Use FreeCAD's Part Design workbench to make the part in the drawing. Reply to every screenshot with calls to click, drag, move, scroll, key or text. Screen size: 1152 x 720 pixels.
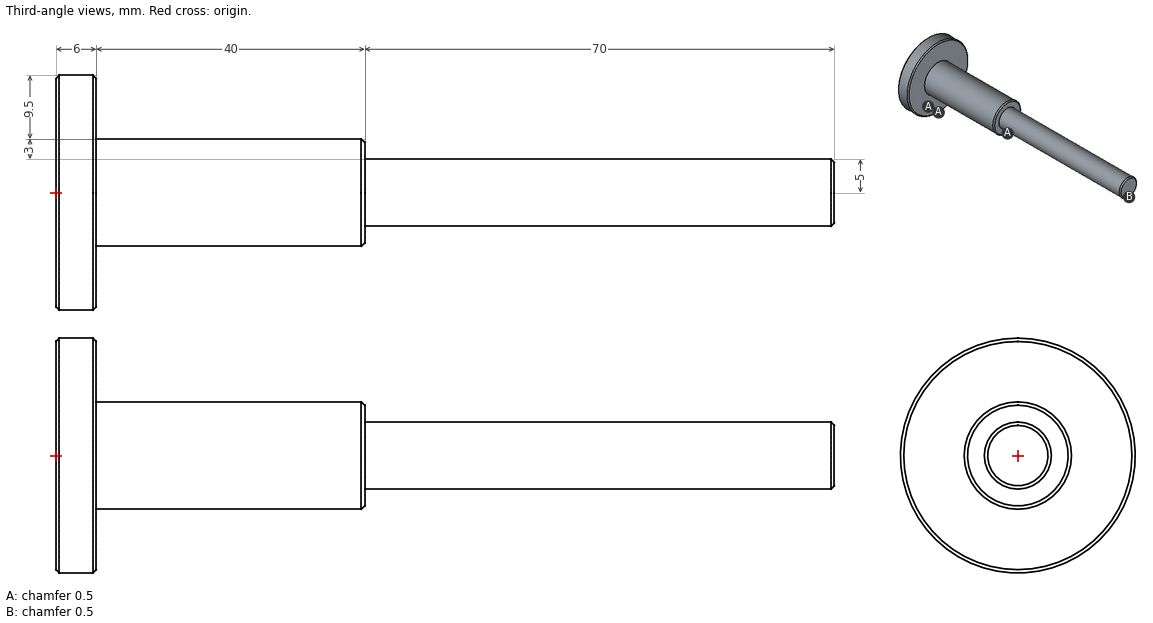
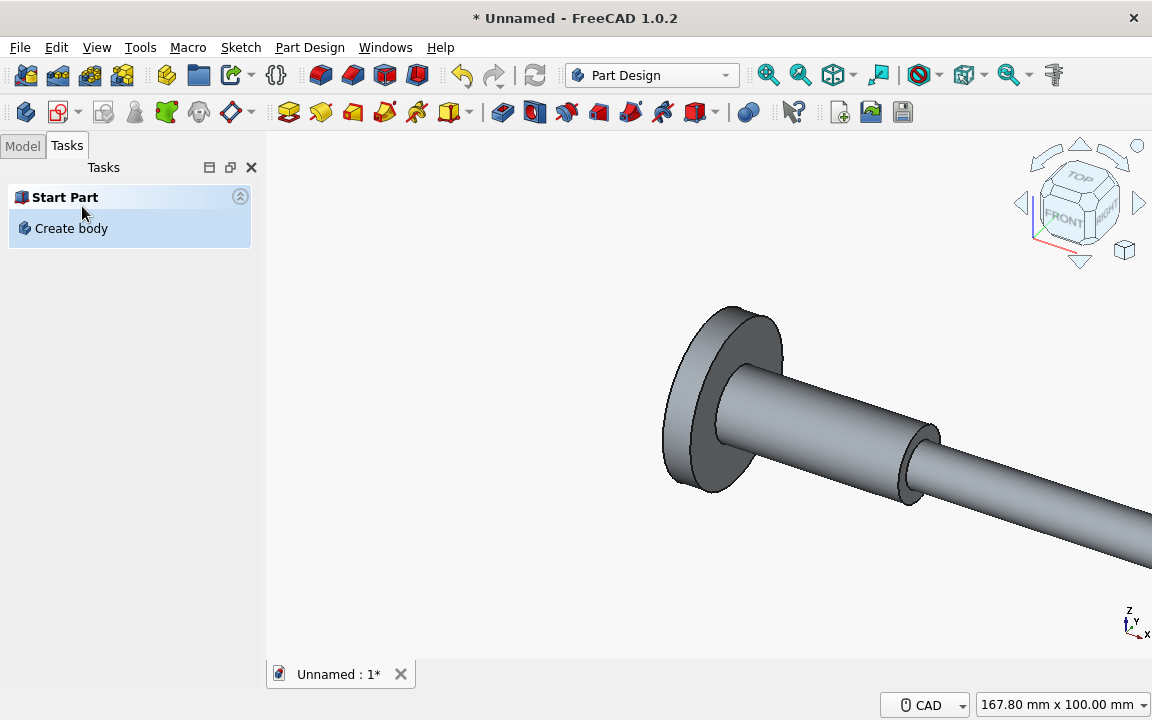
click(770, 76)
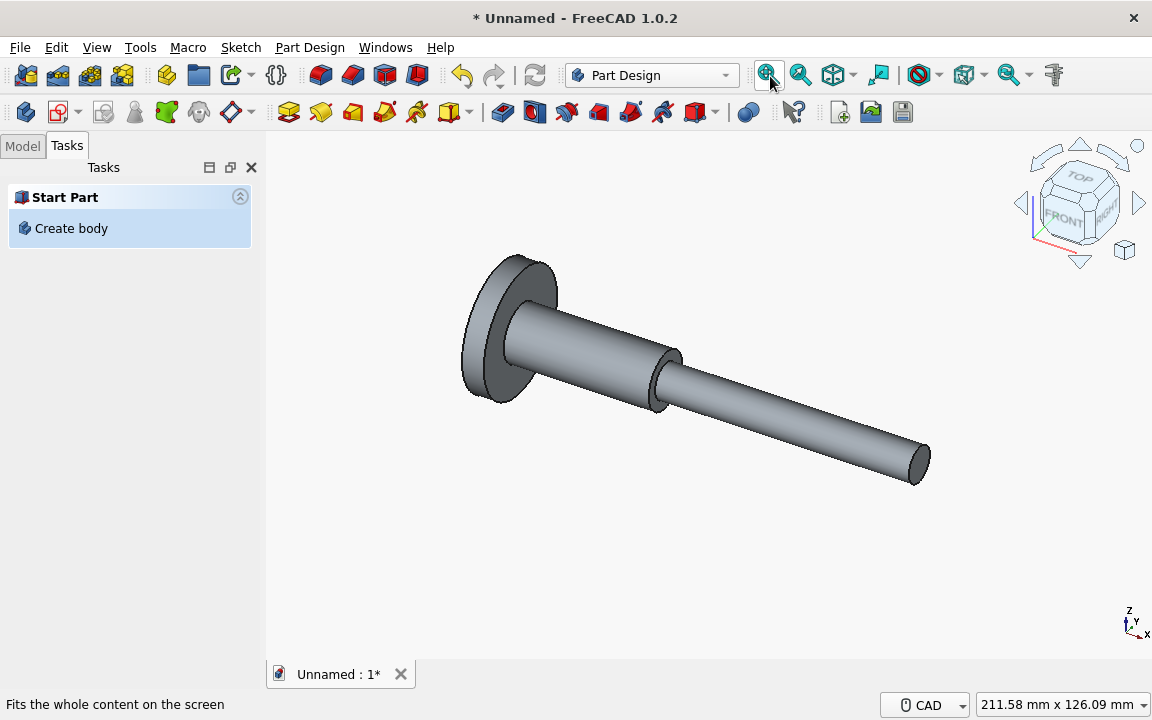
click(649, 396)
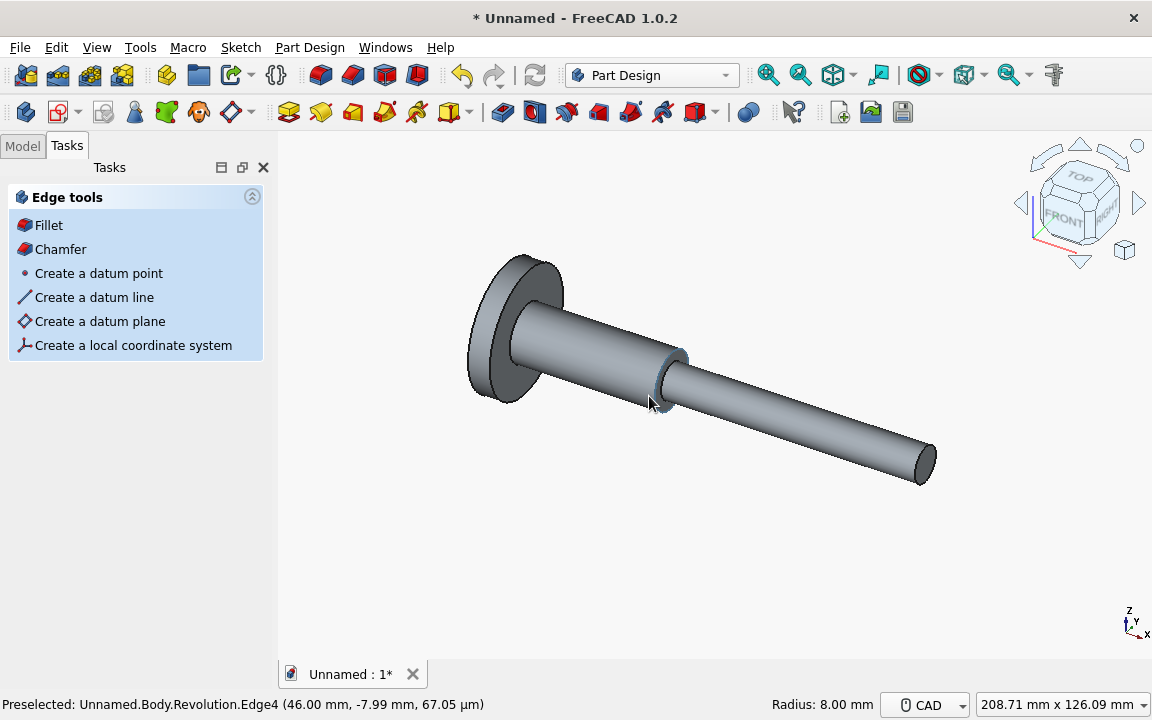
click(490, 368, ctrl)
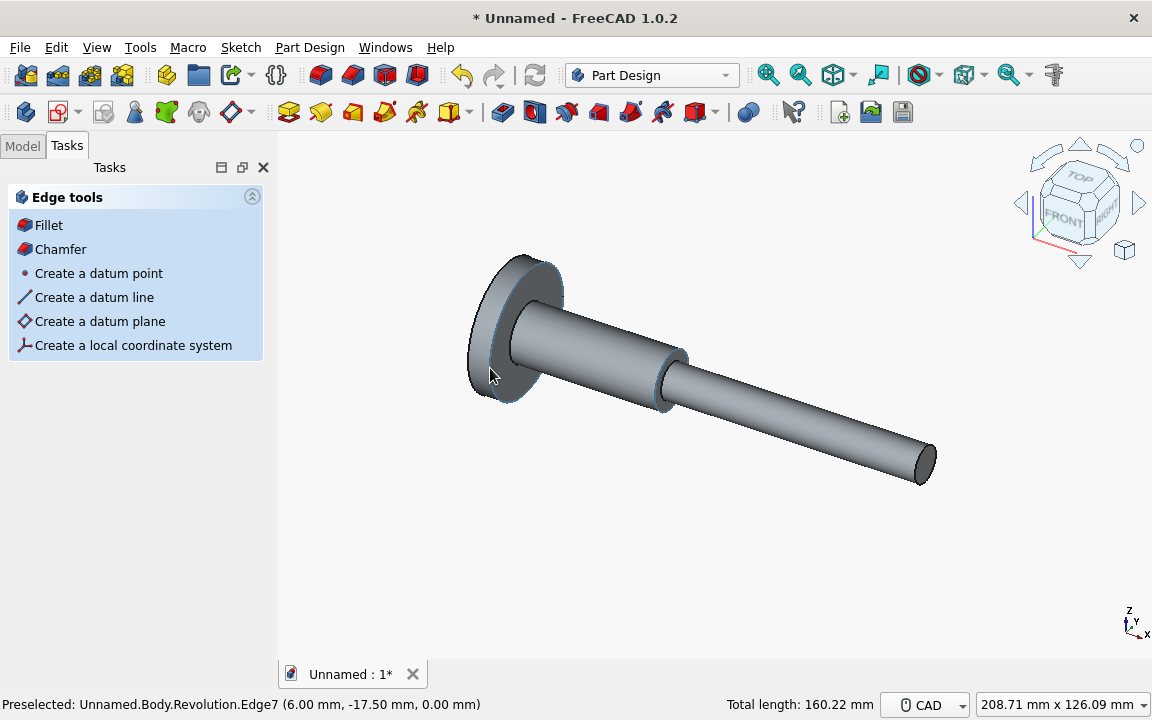
key(0)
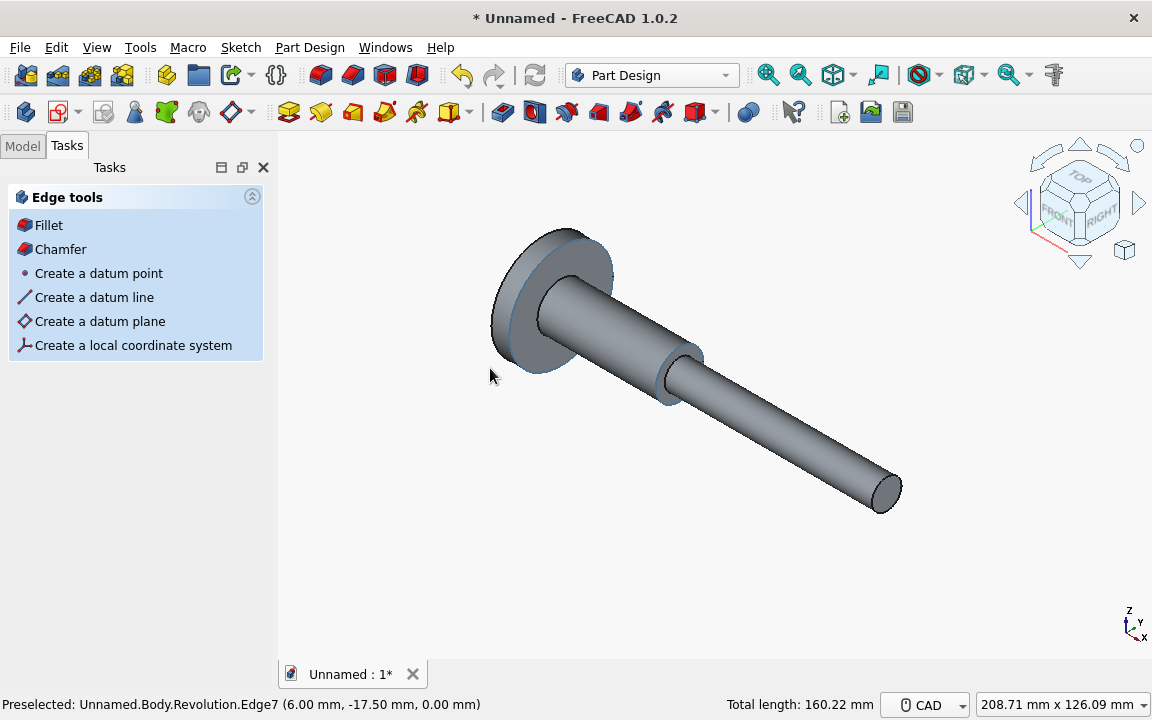
key(2)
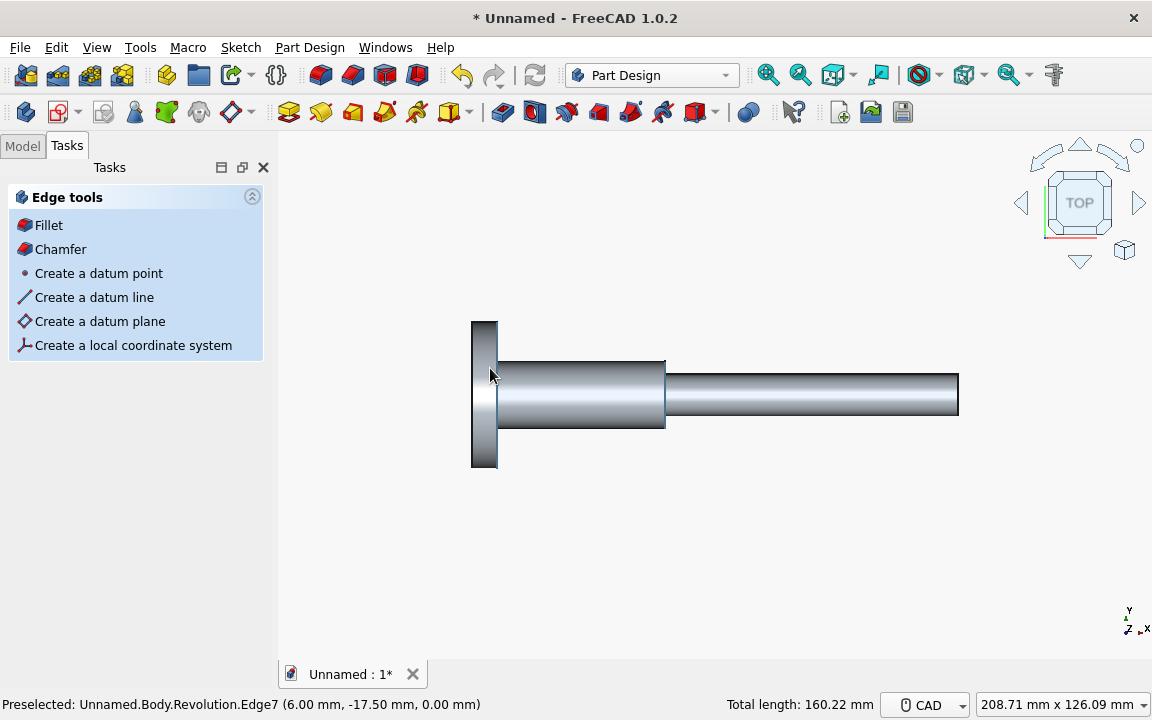
click(472, 453, ctrl)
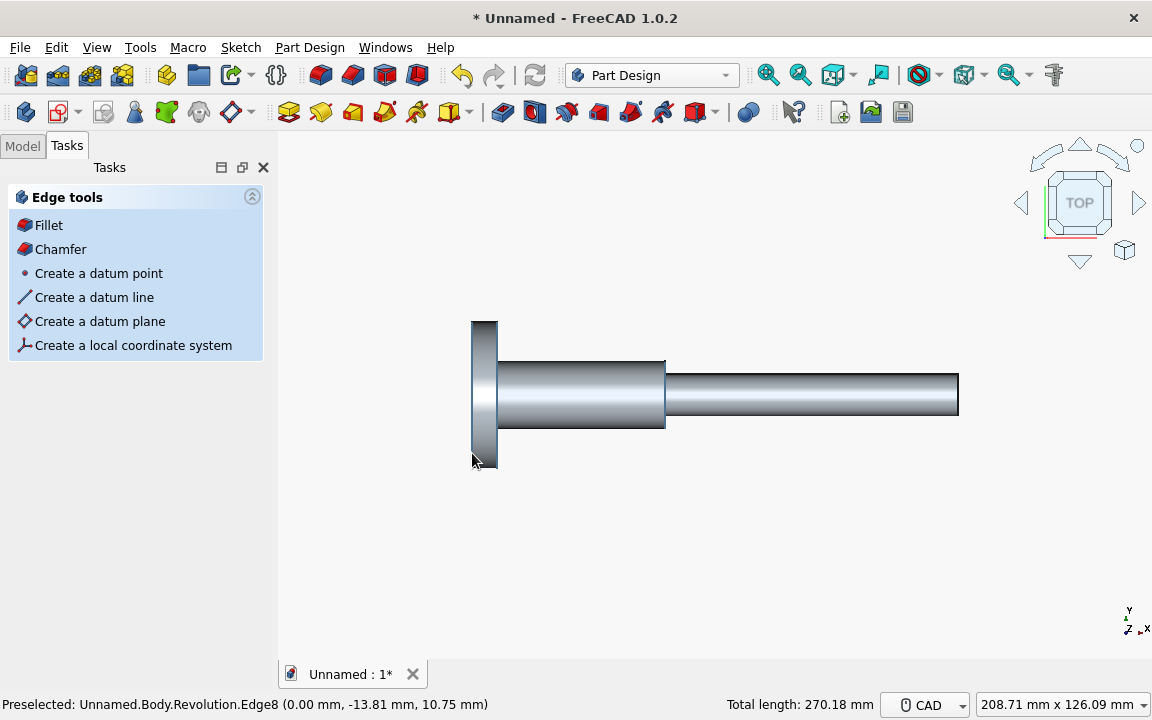
click(354, 76)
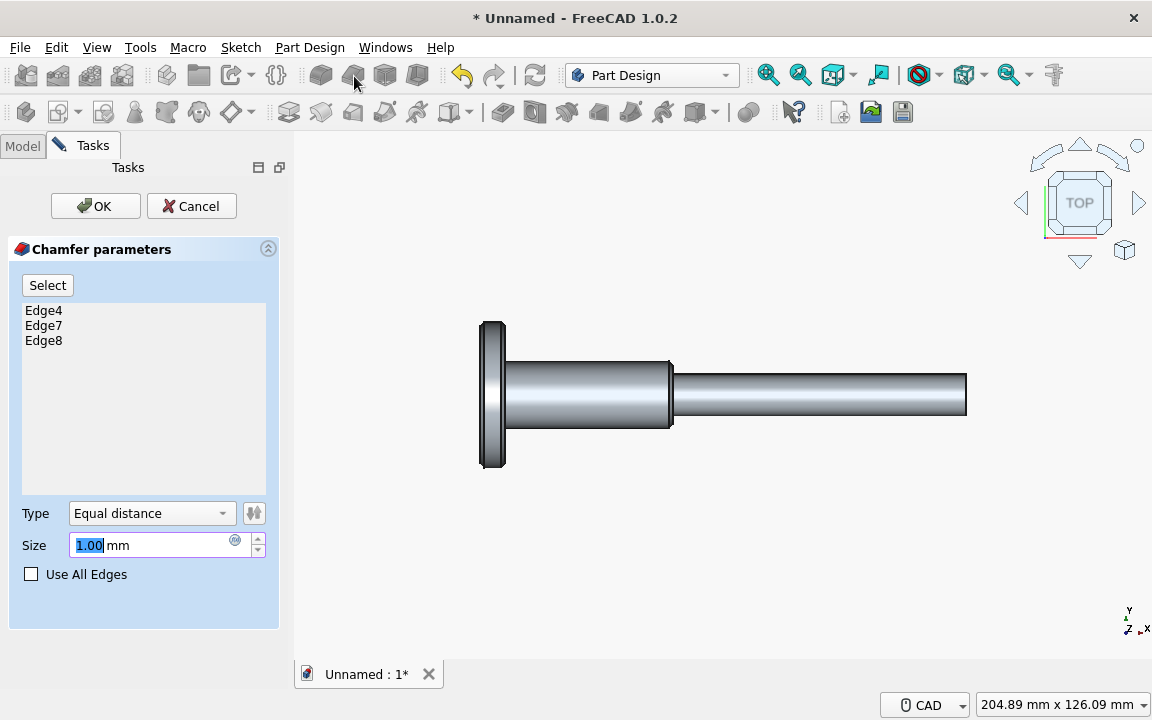
text(0.5)
key(Tab)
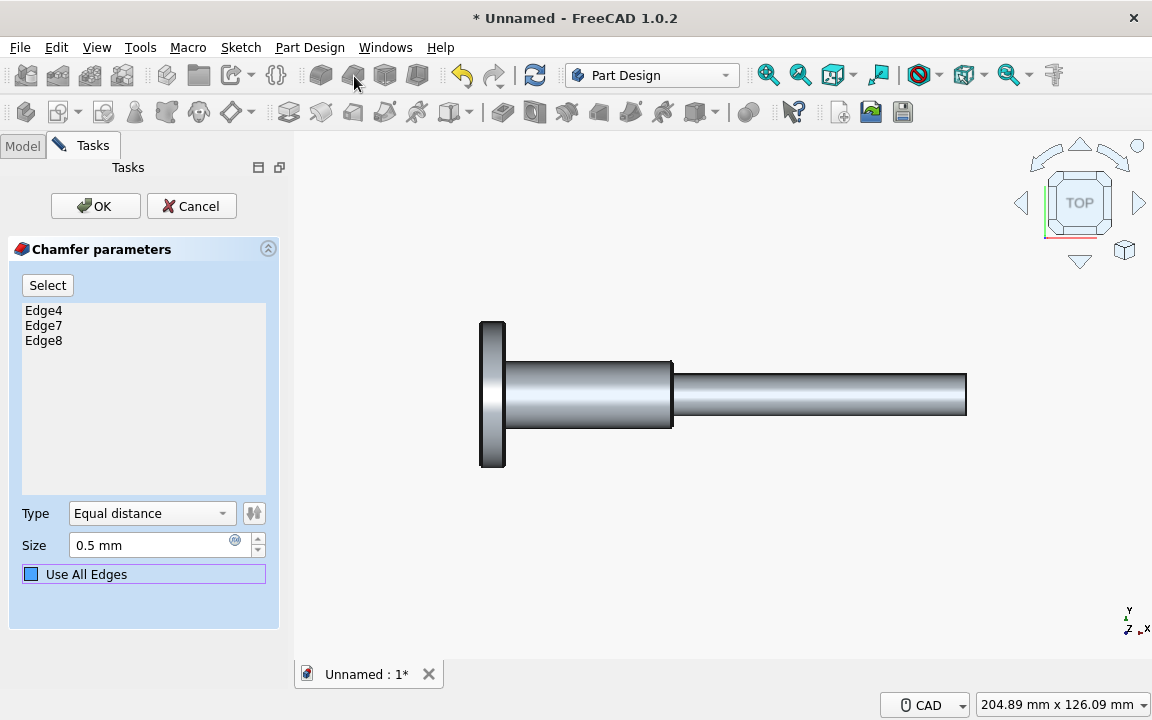
click(96, 206)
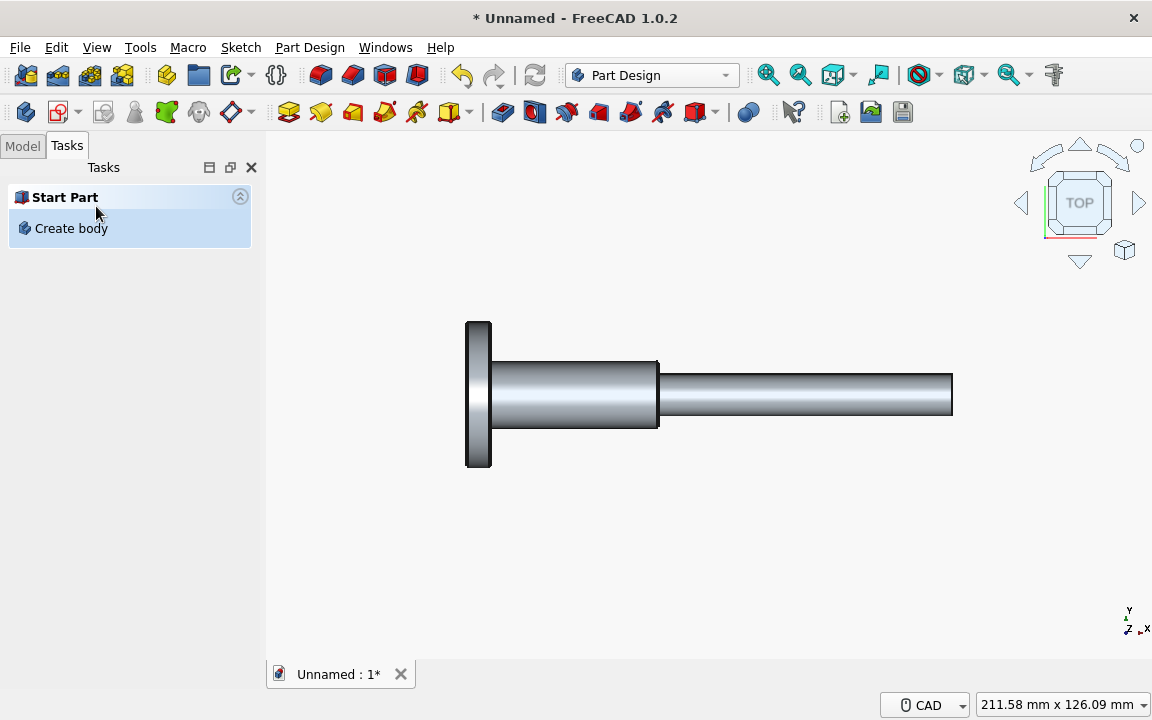
click(952, 415)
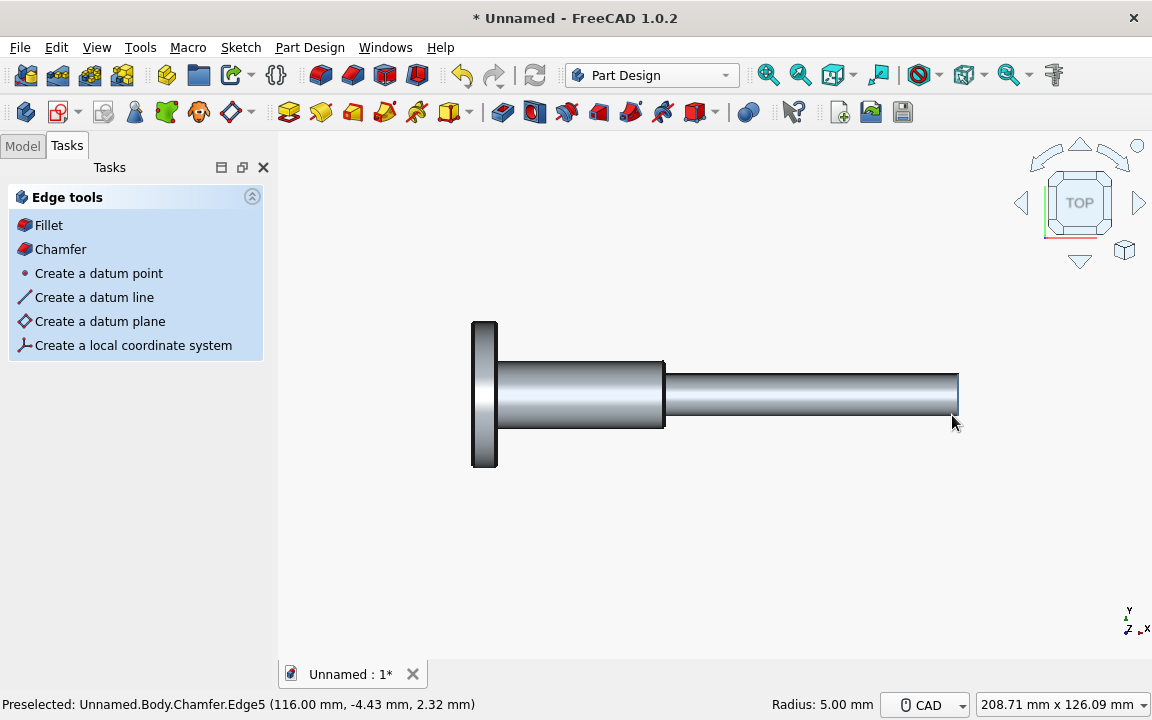
click(354, 76)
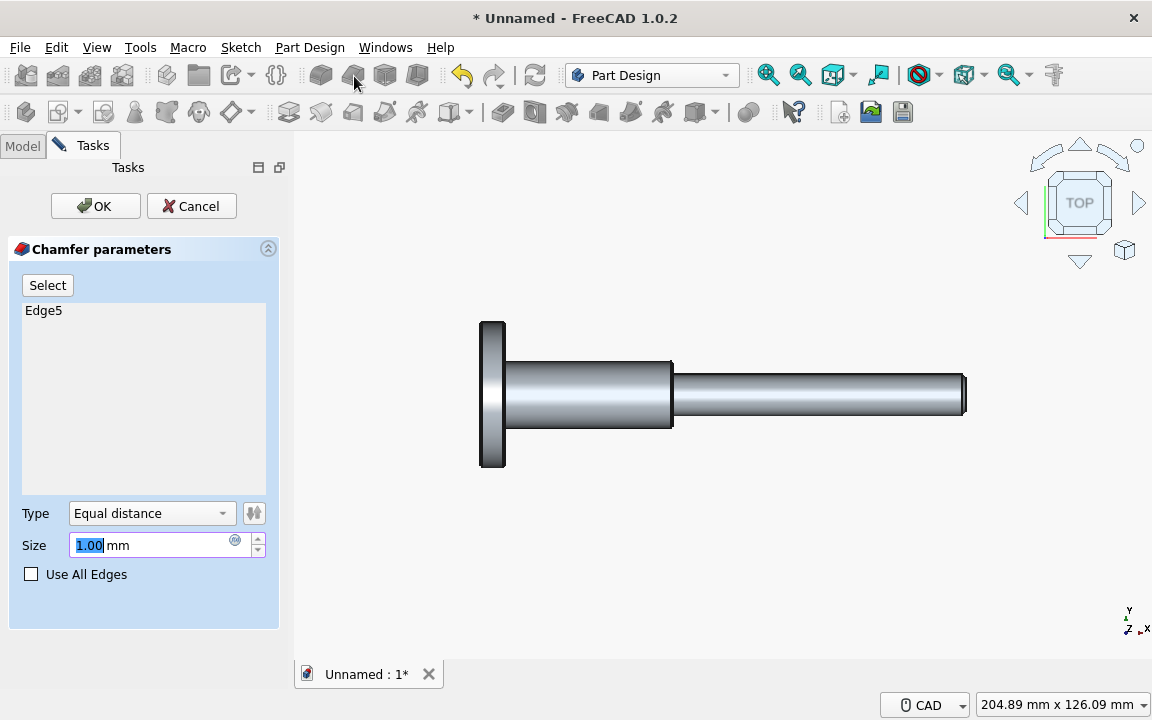
text(0.5)
key(Tab)